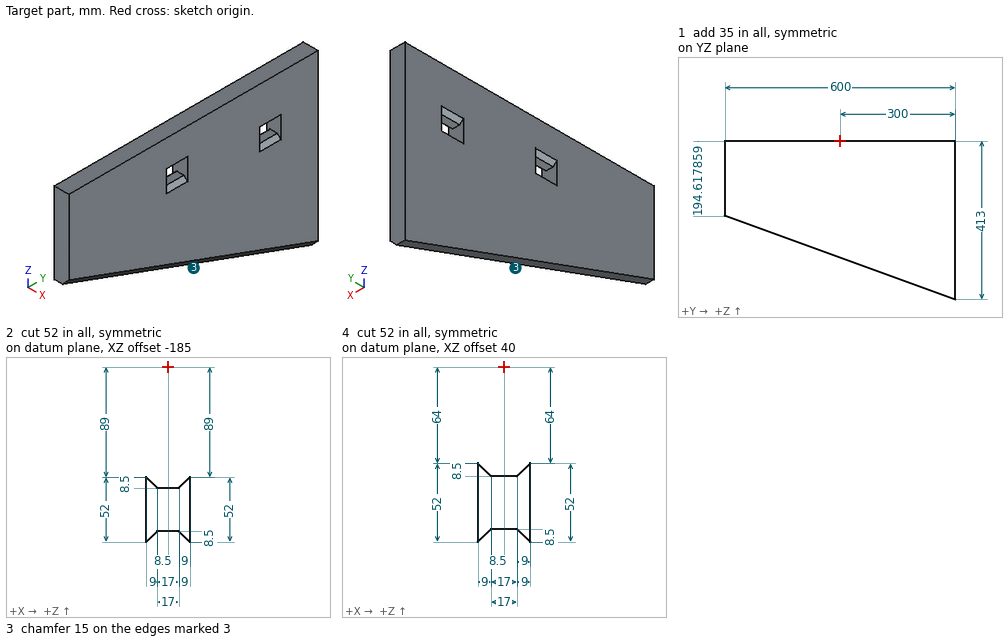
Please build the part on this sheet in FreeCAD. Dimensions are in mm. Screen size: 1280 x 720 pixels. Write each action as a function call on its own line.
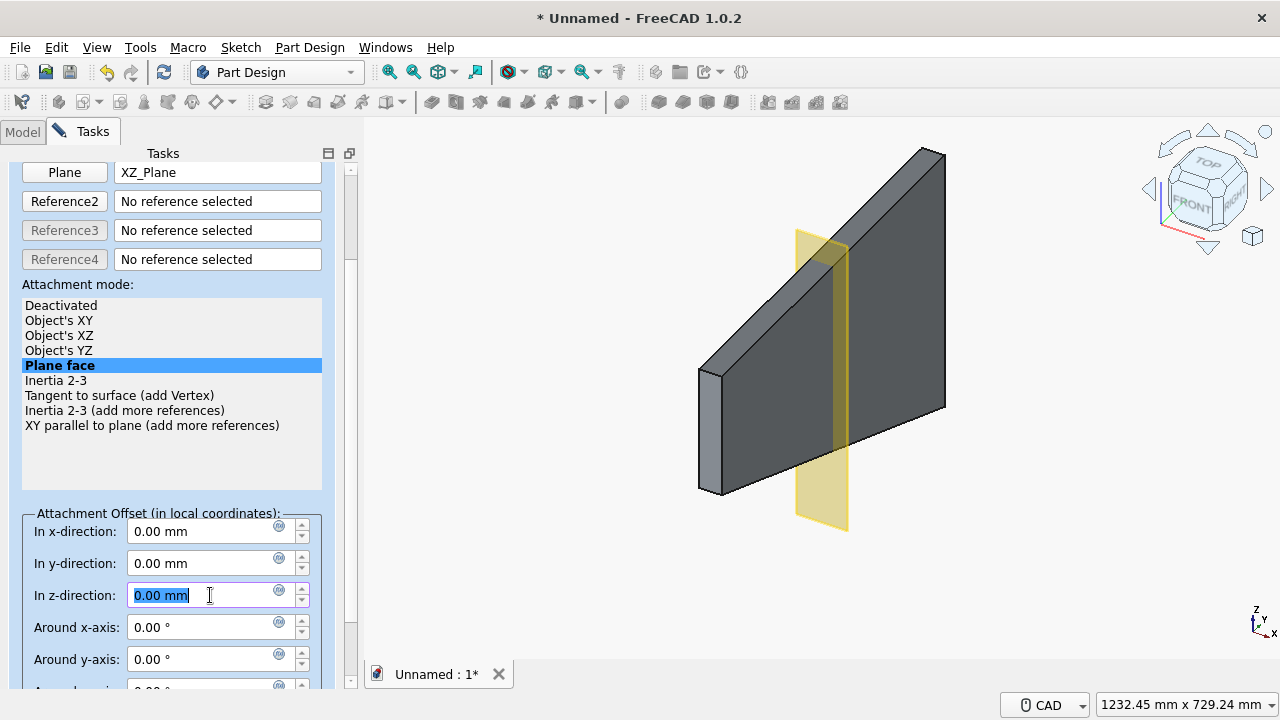
text(-185)
key(Tab)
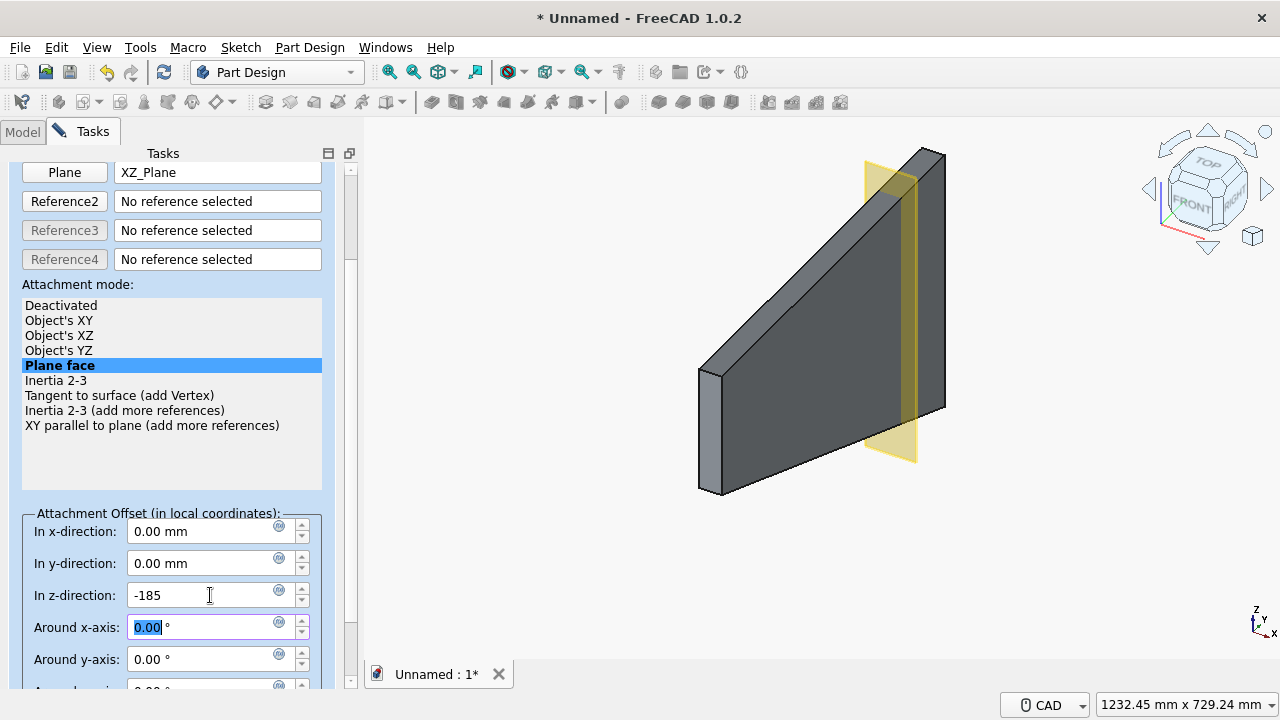
scroll(351, 426, up, 3)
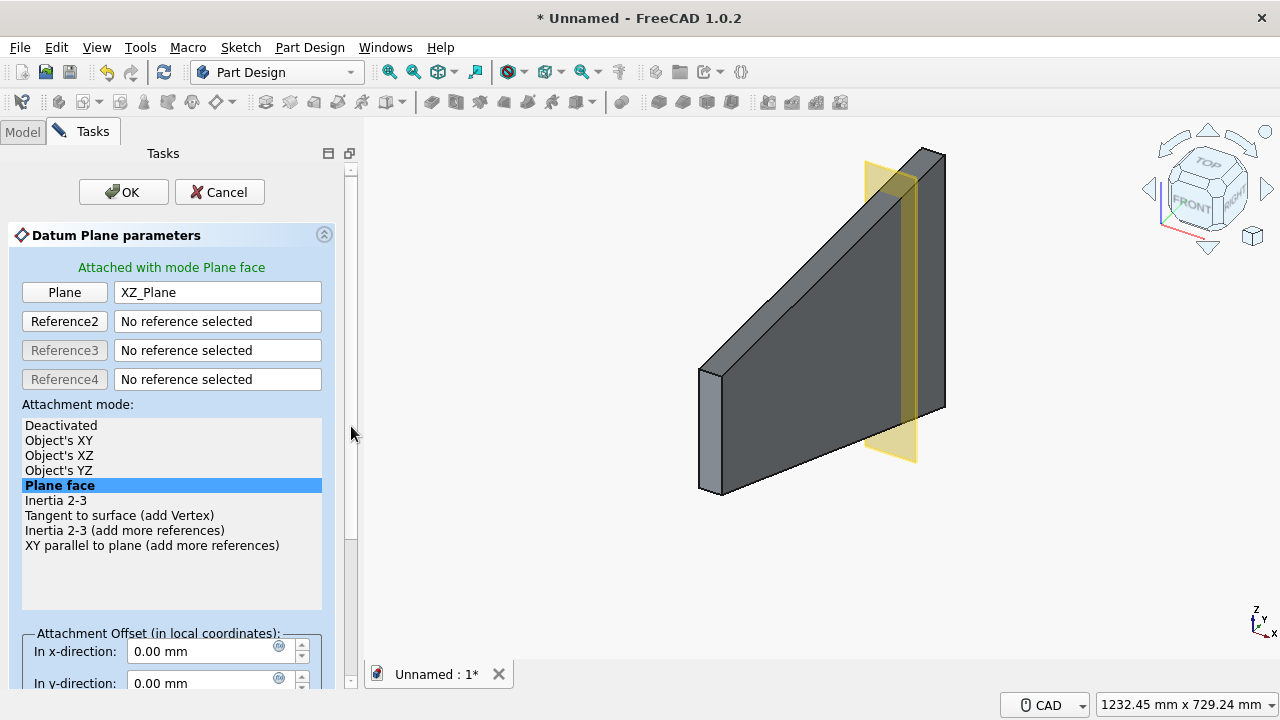
click(124, 192)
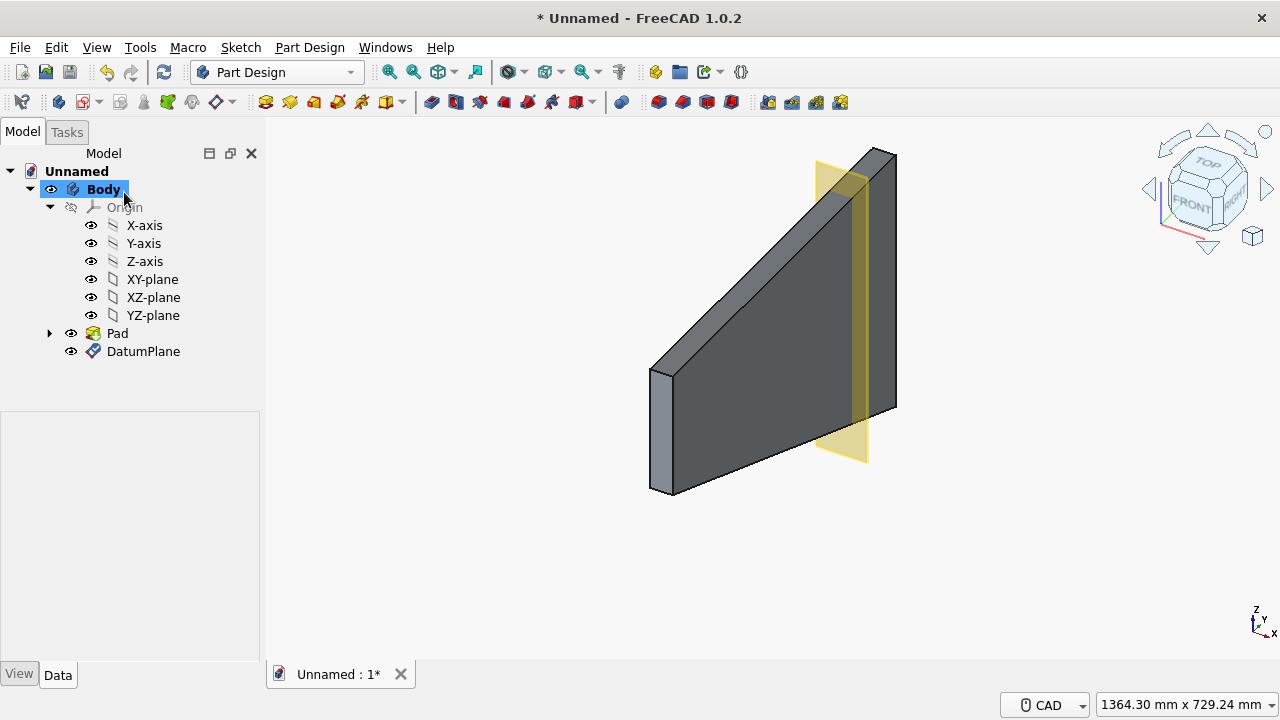
click(116, 351)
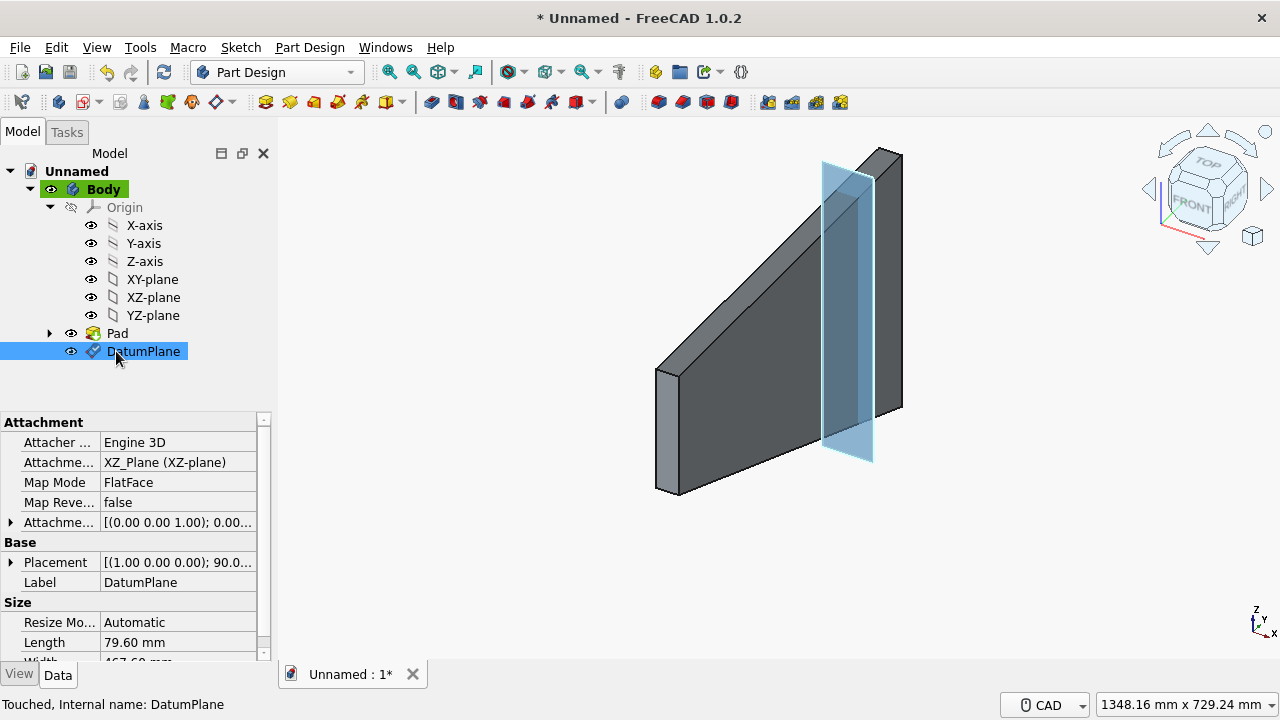
click(84, 102)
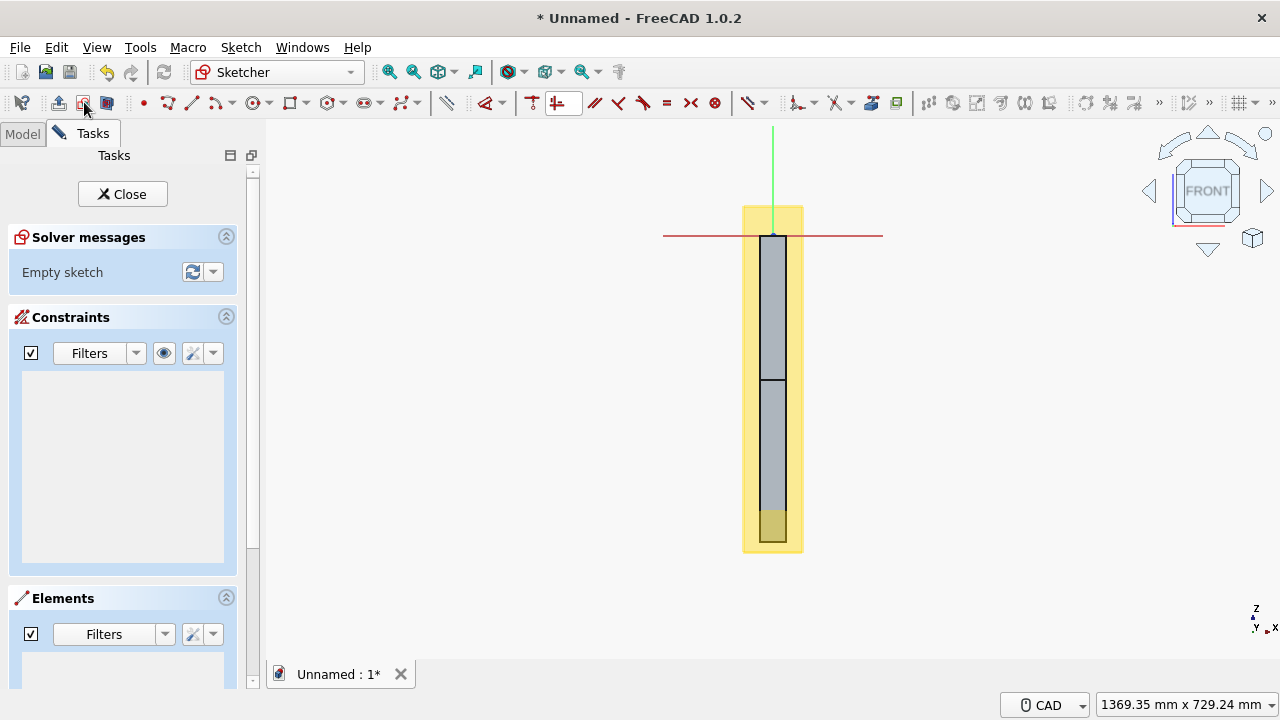
key(q)
key(s)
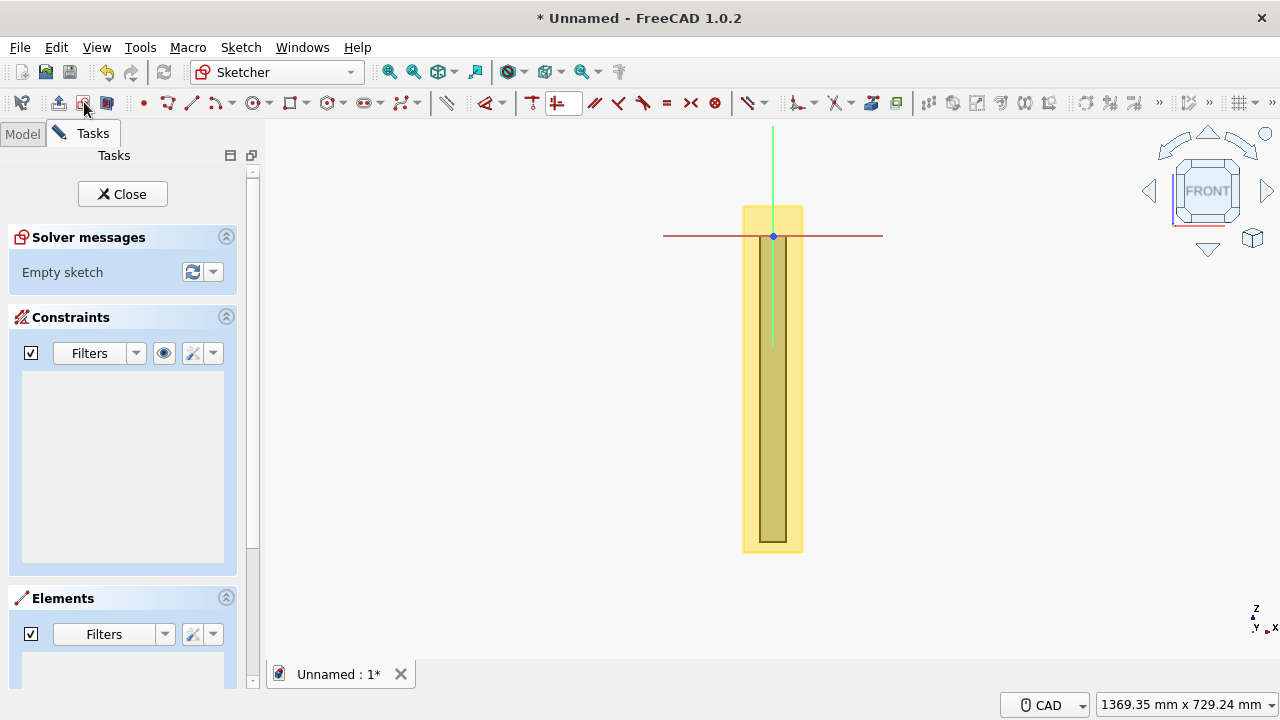
scroll(782, 313, up, 11)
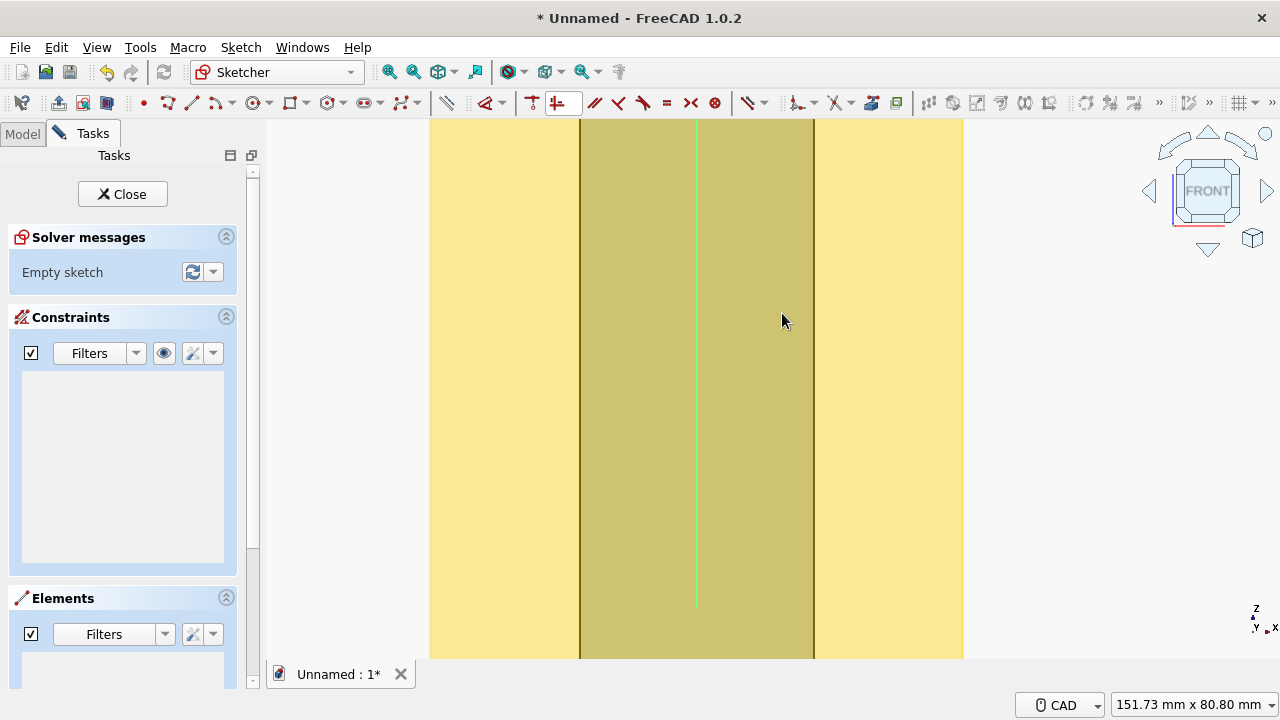
key(g)
key(m)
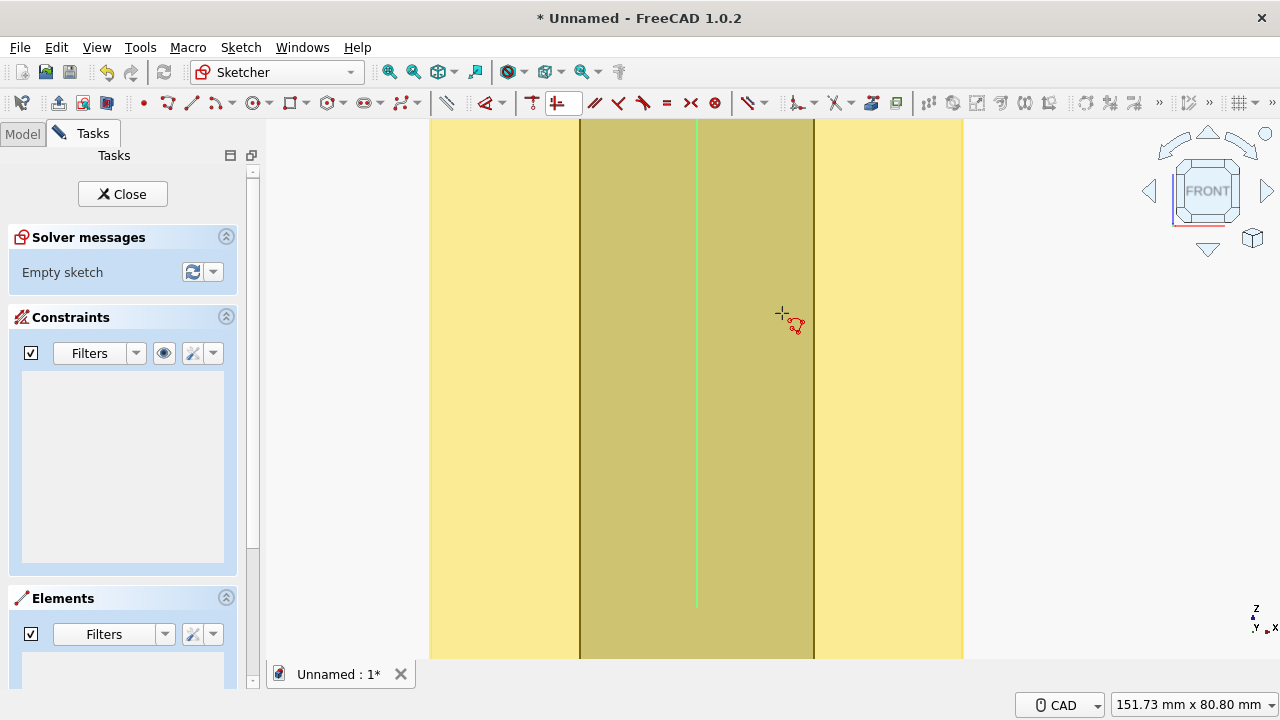
click(580, 211)
click(640, 268)
click(753, 268)
click(814, 211)
click(814, 558)
click(753, 501)
click(640, 501)
click(580, 558)
click(580, 212)
key(Escape)
key(Escape)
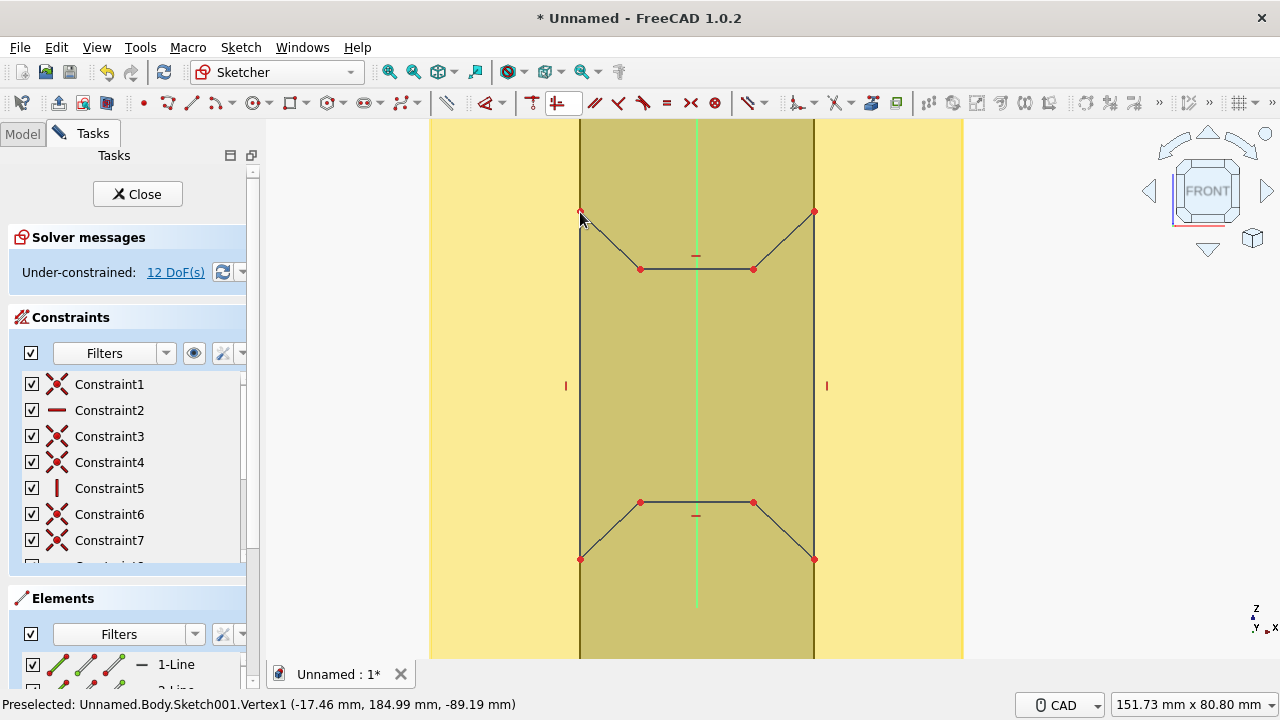
click(674, 269)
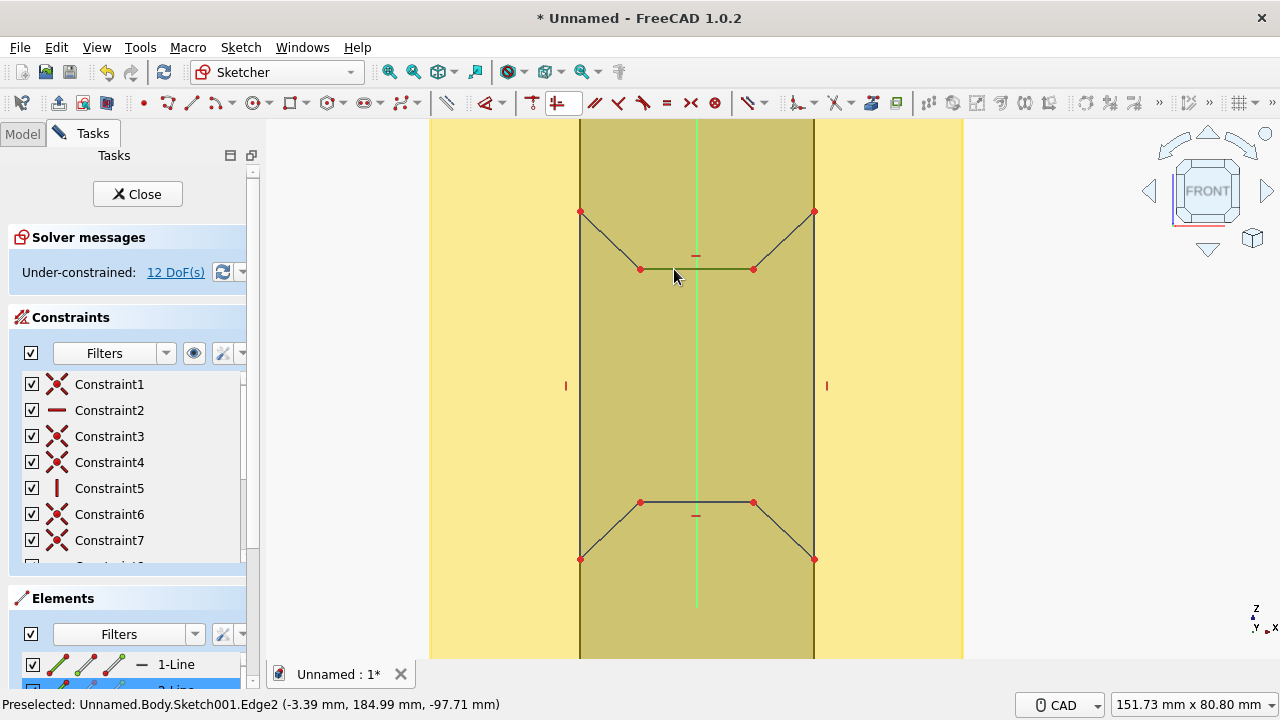
key(l)